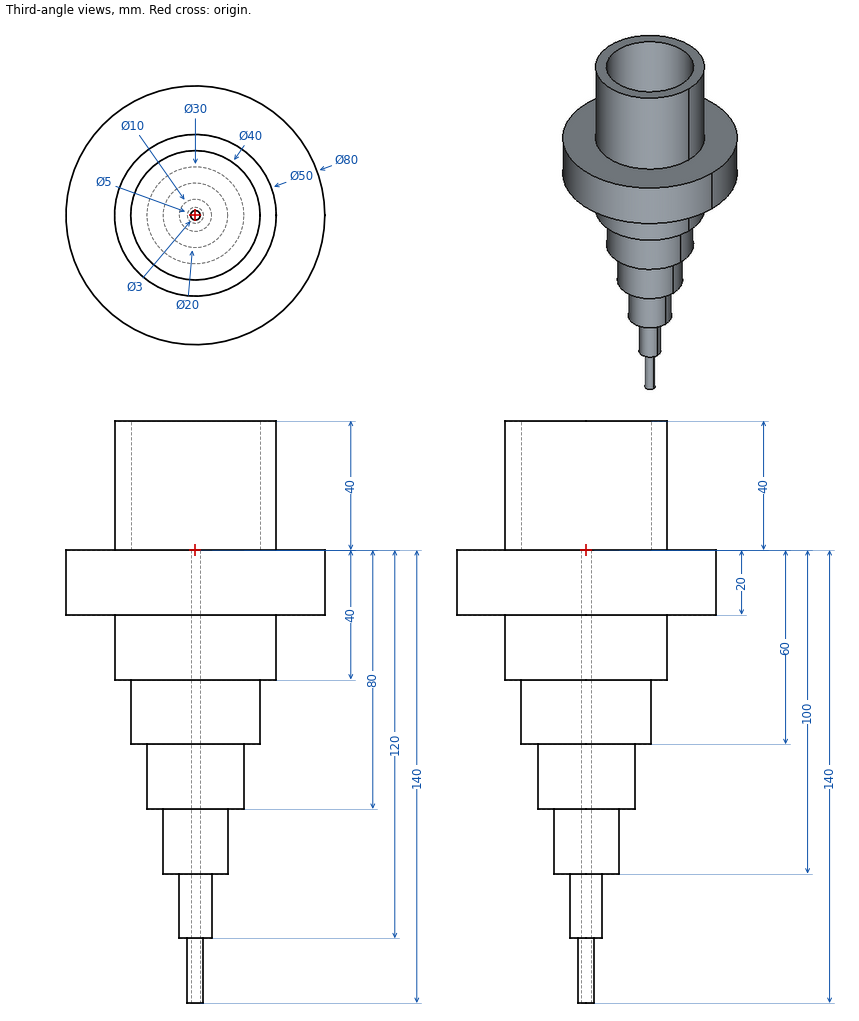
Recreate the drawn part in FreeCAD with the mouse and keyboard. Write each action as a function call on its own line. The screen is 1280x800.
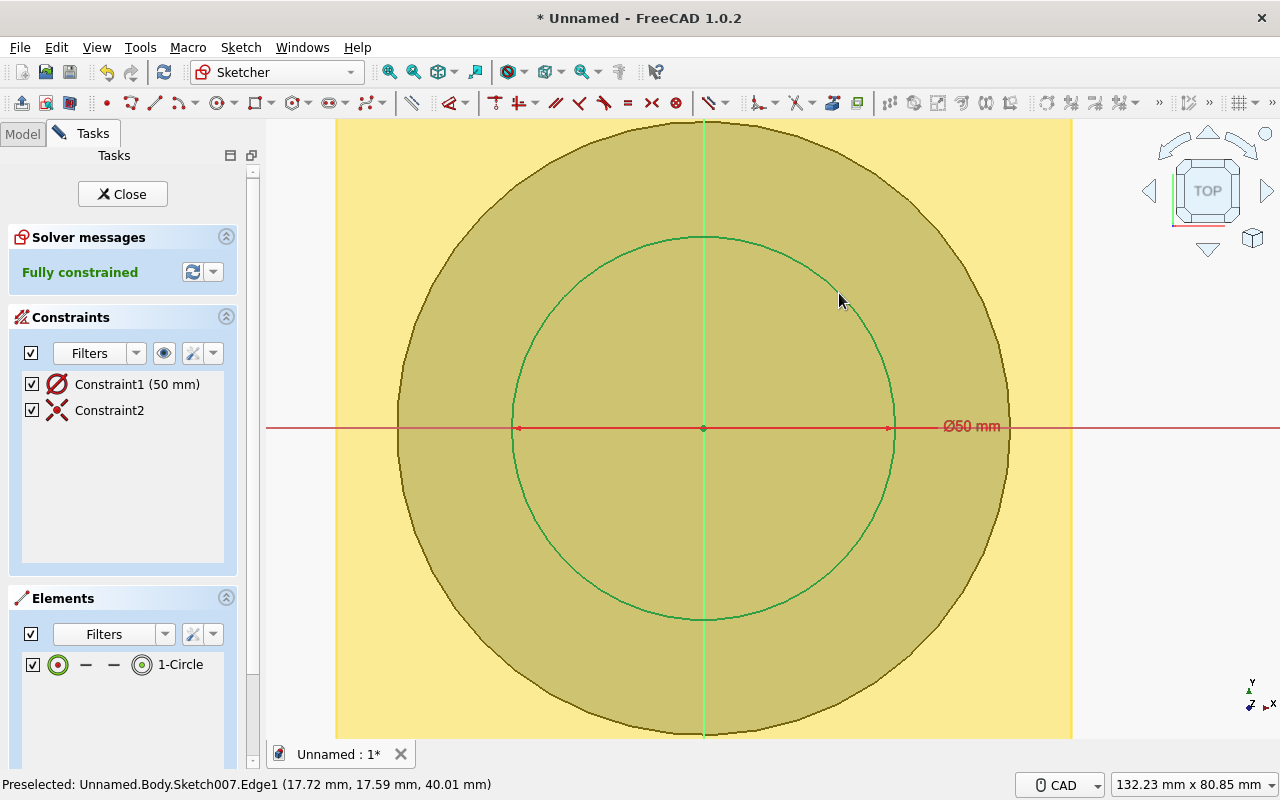
click(123, 194)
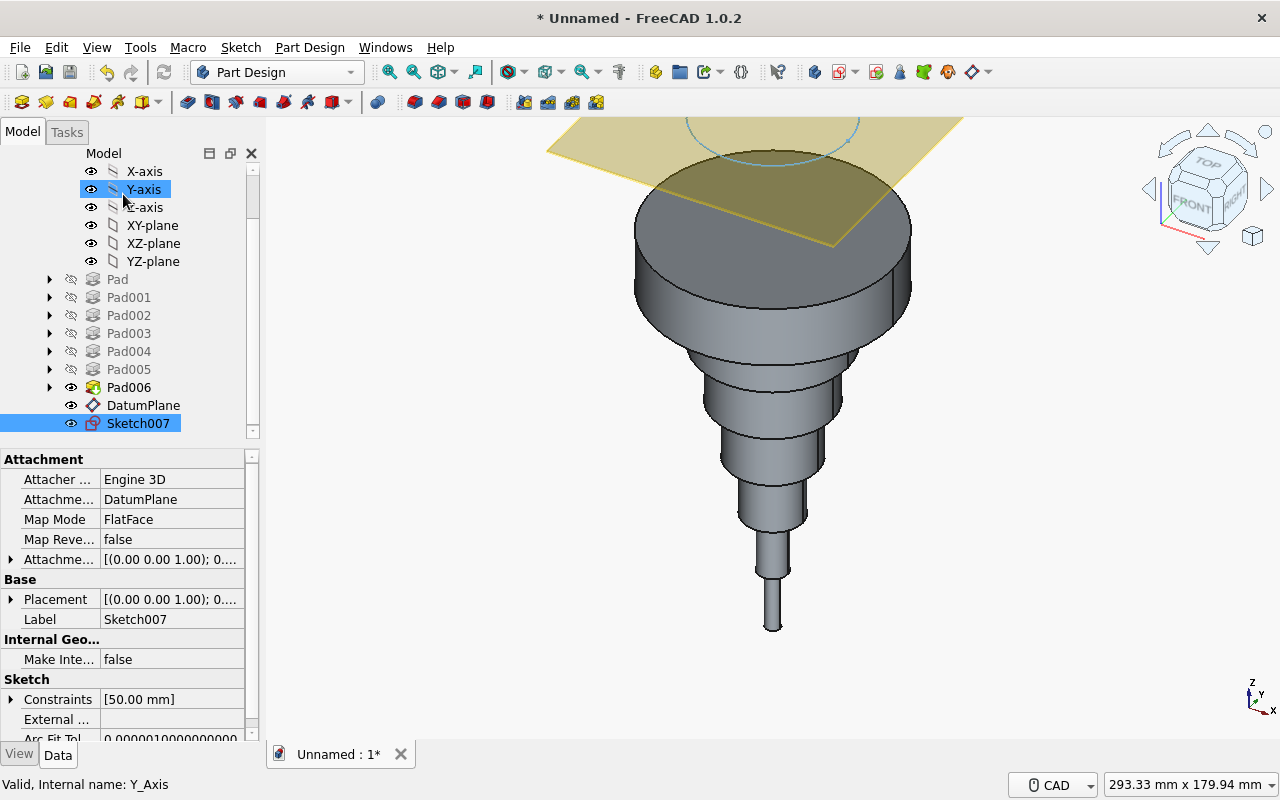
click(22, 102)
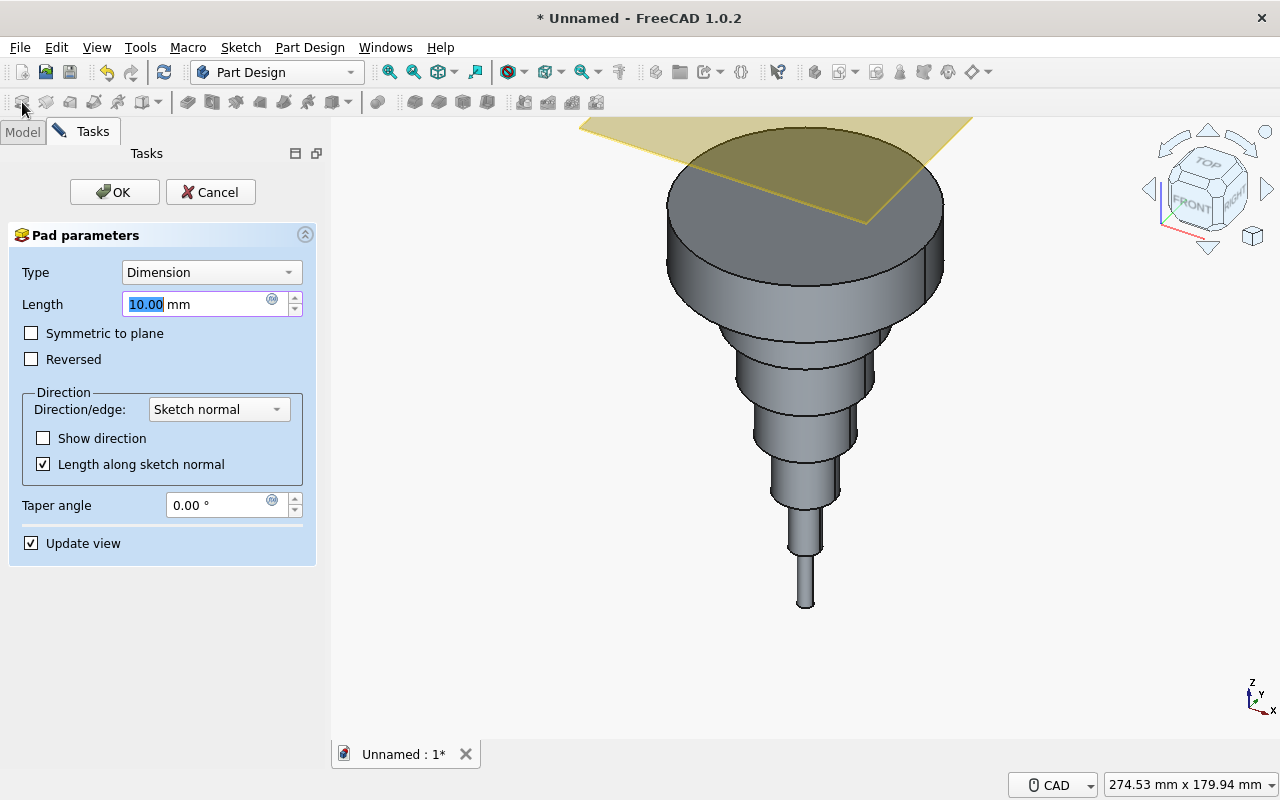
text(40)
key(Tab)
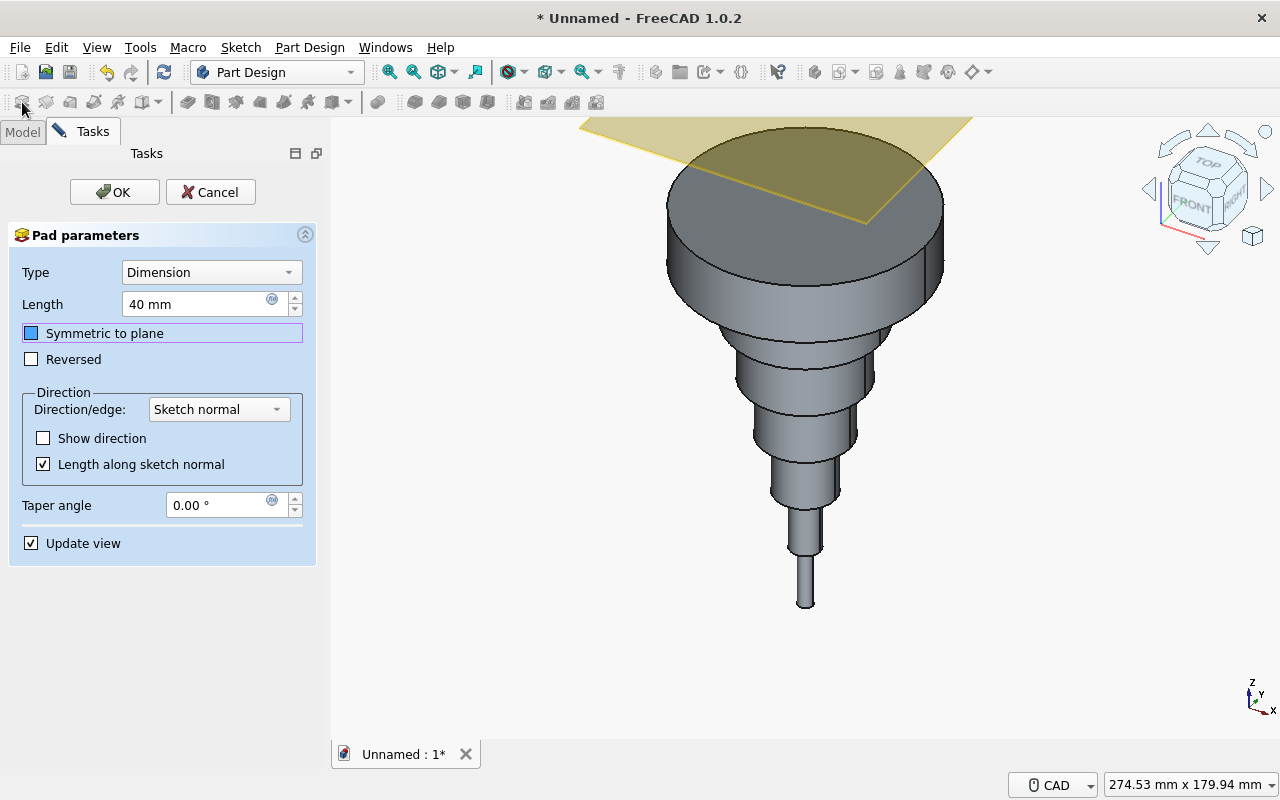
click(30, 359)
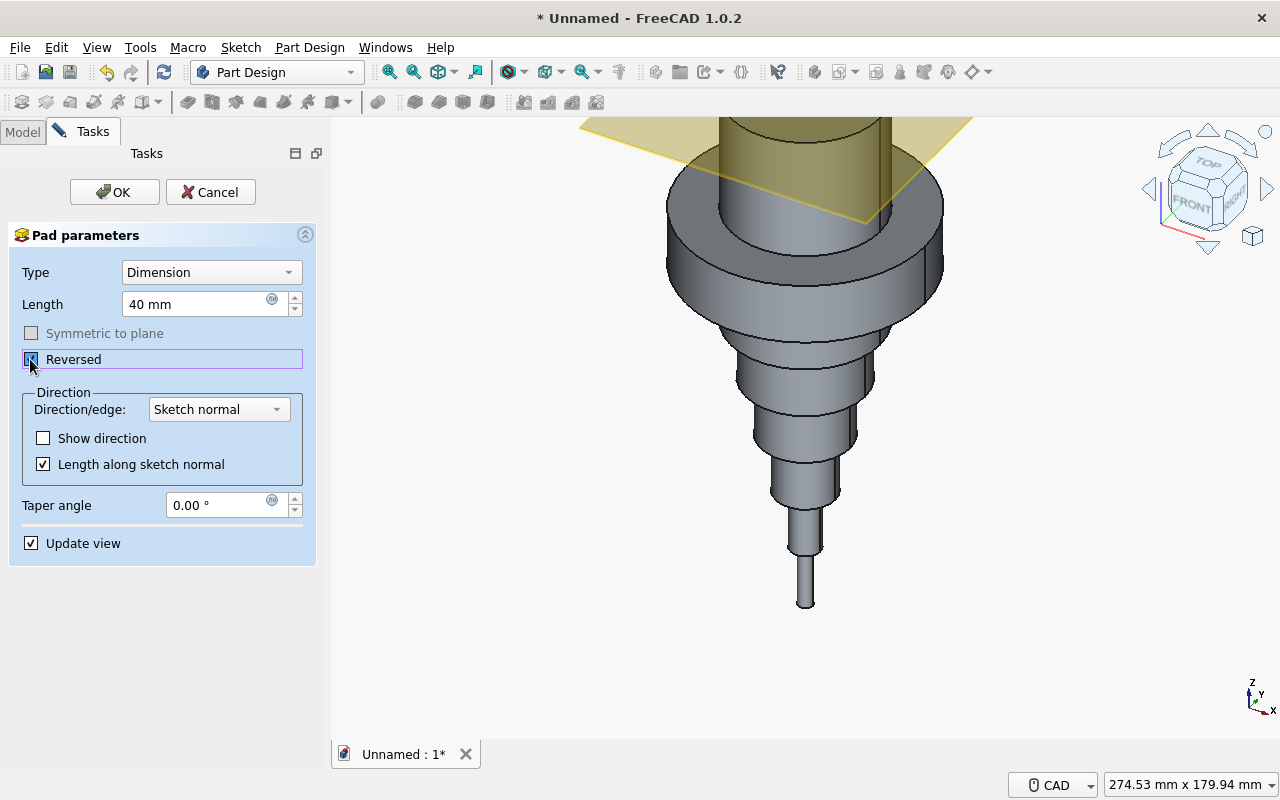
click(115, 192)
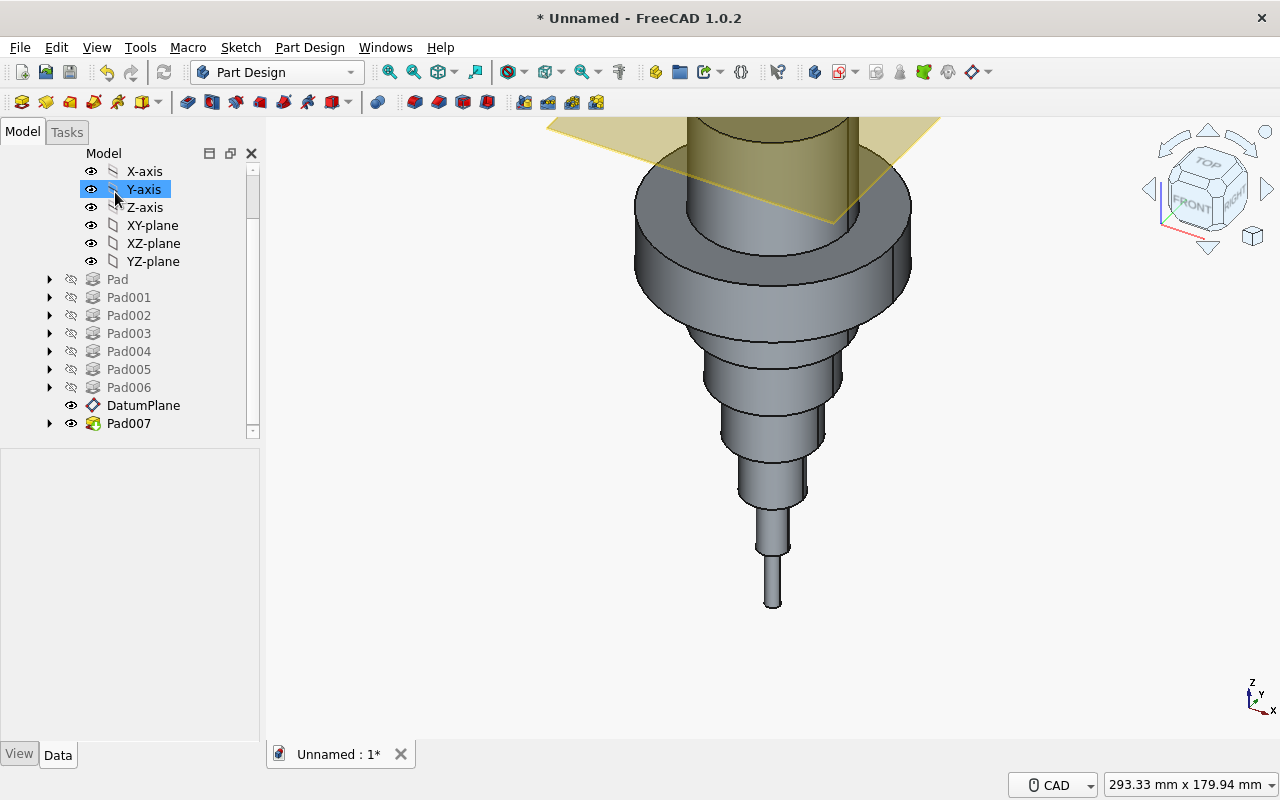
click(116, 405)
key(space)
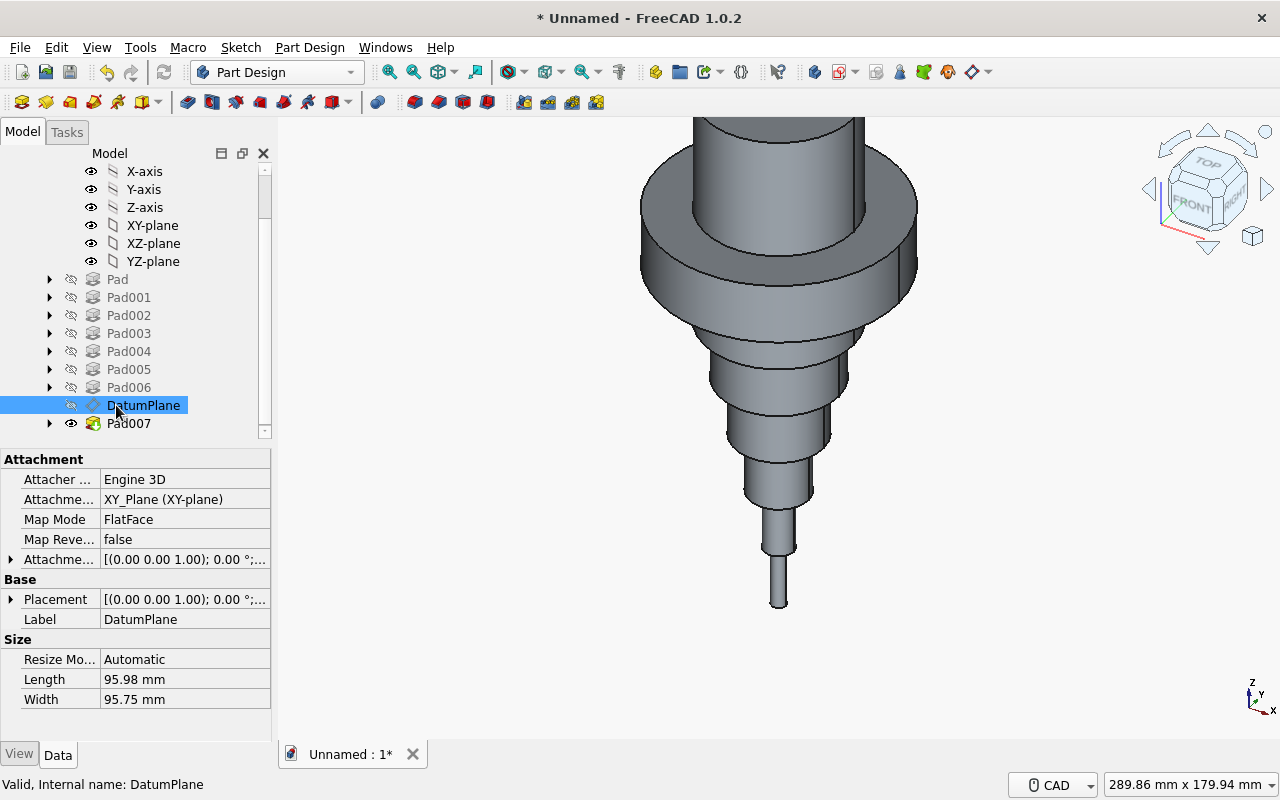
click(390, 72)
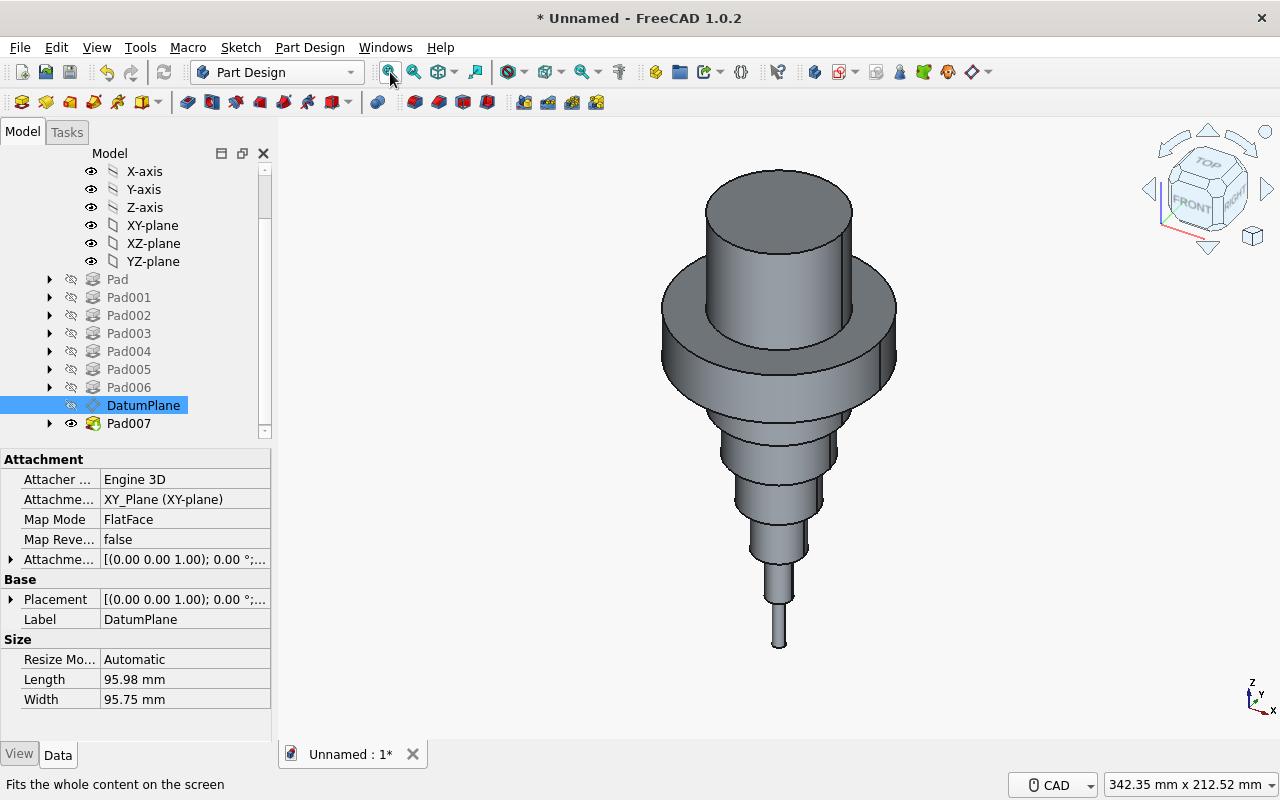
click(779, 211)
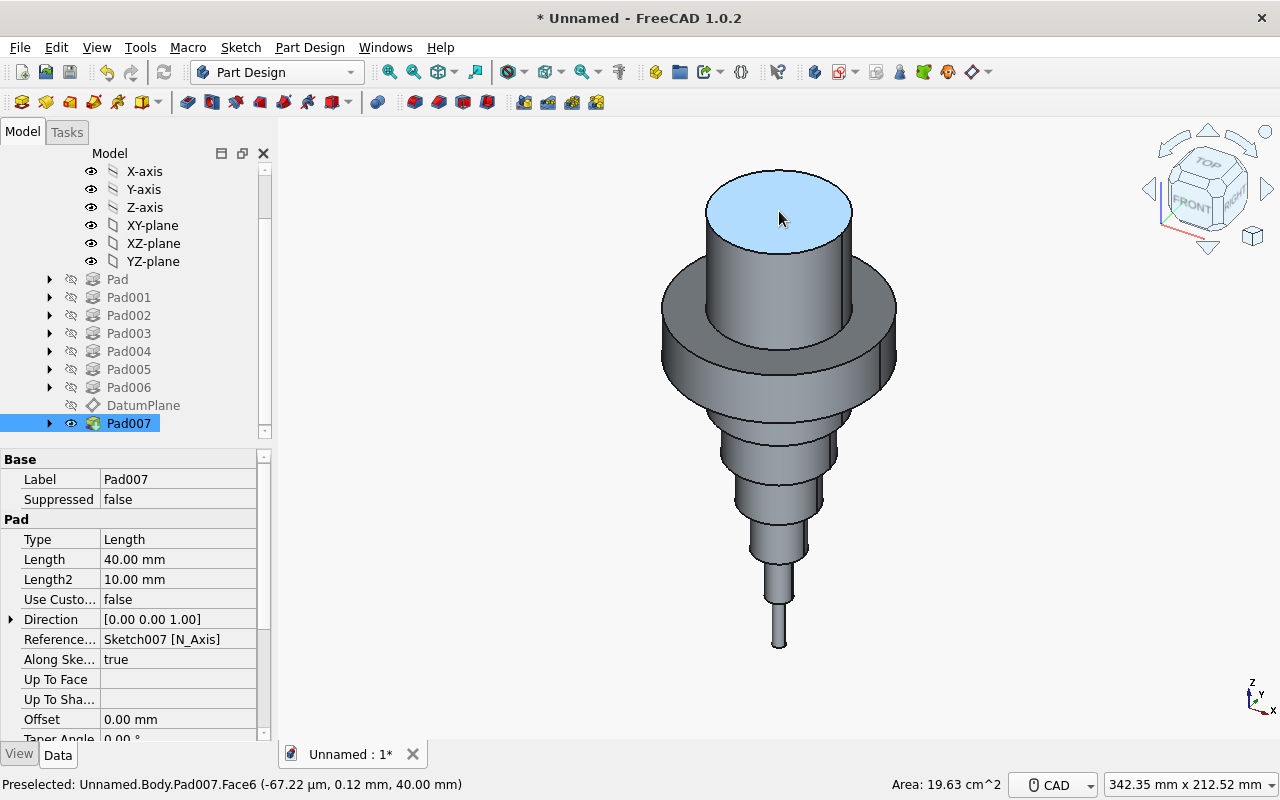
click(840, 72)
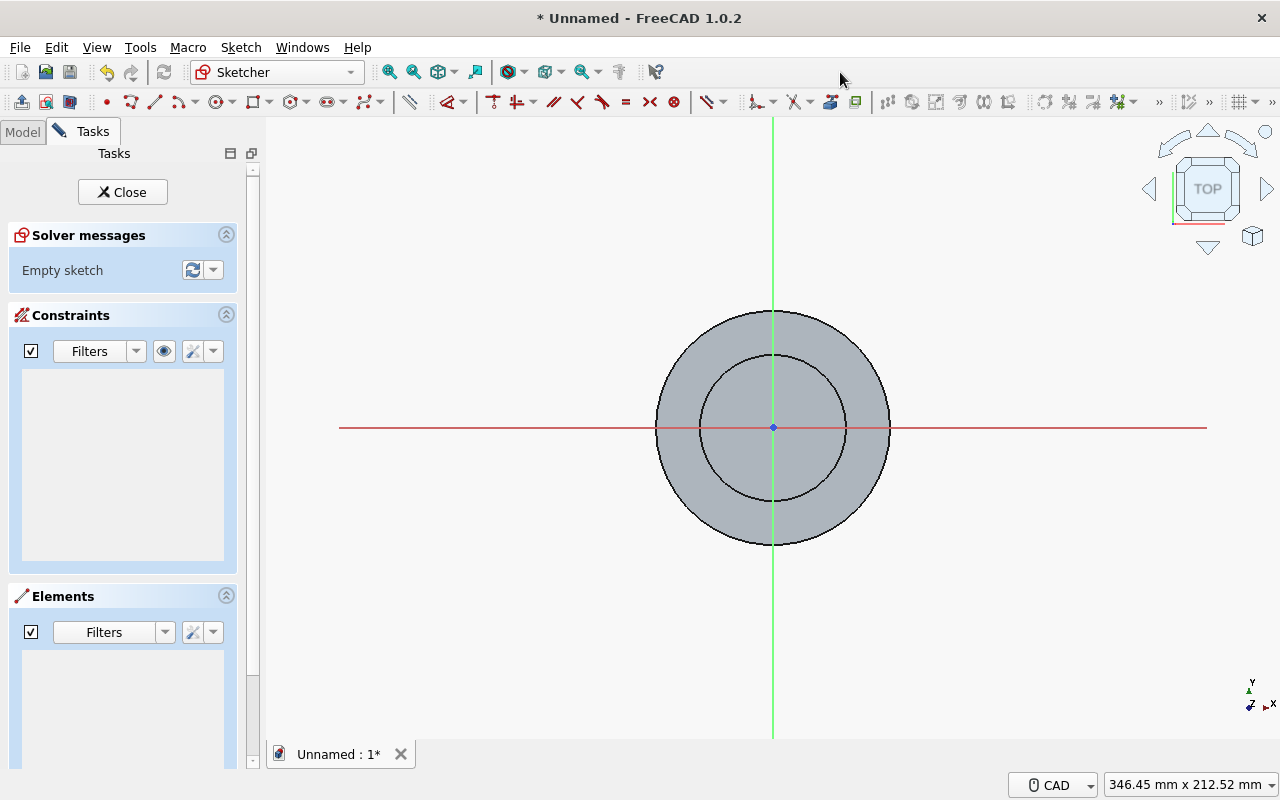
scroll(803, 428, up, 6)